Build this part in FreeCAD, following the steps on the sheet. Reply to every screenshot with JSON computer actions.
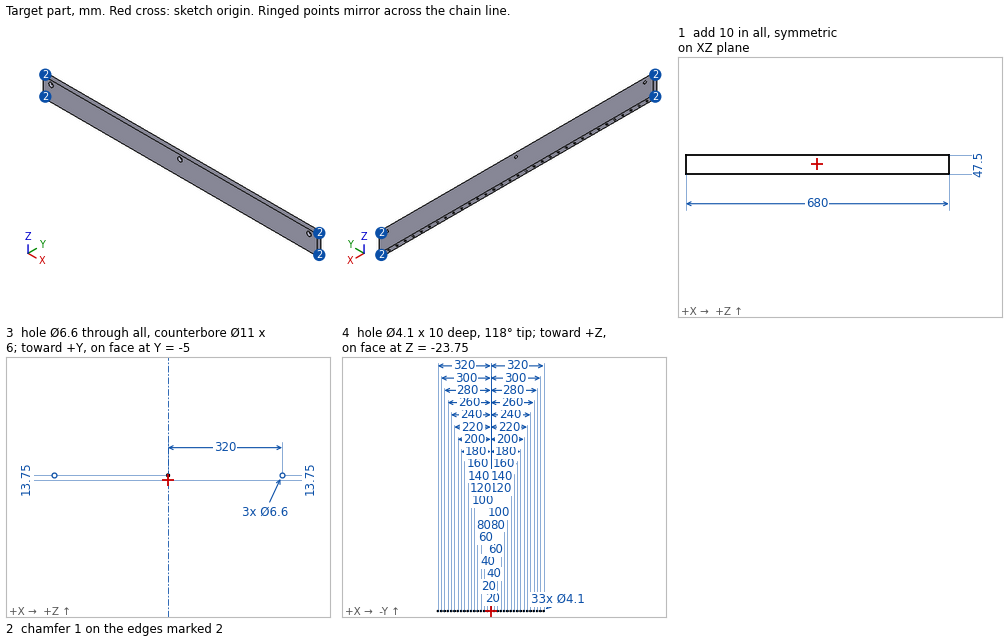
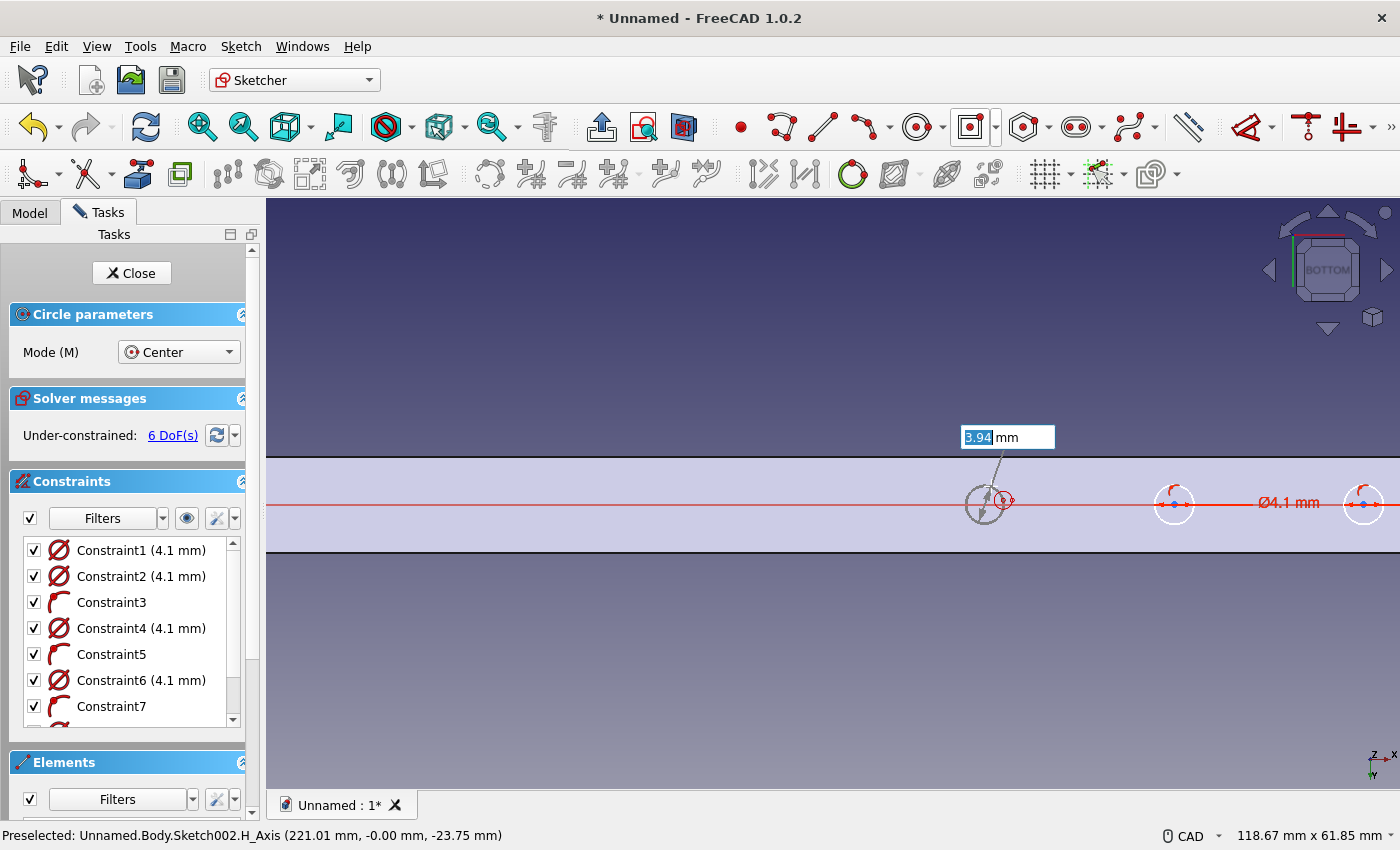
{"action": "type", "text": "4.1"}
{"action": "key", "text": "Return"}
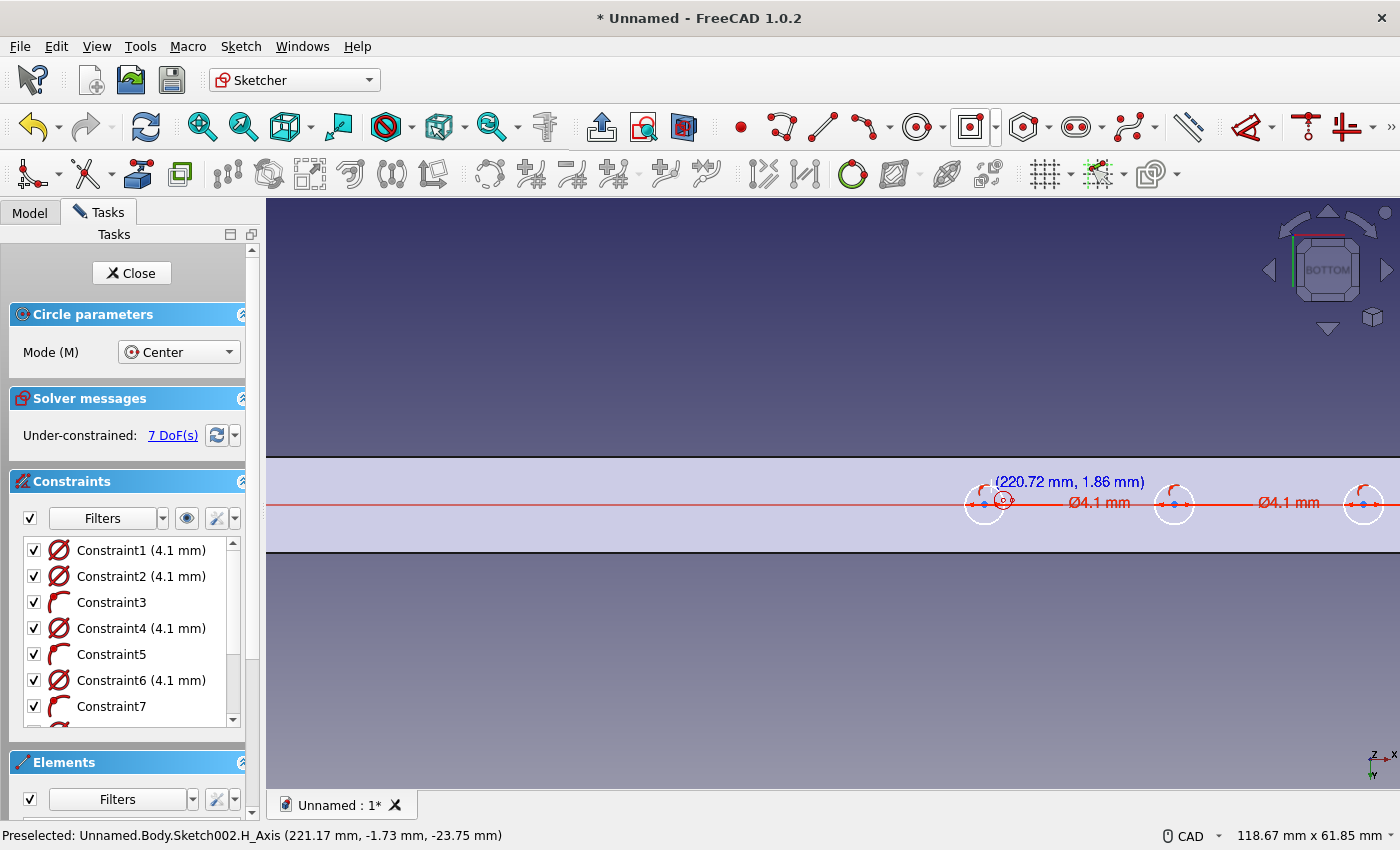
{"action": "scroll", "coordinate": [999, 492], "scroll_direction": "down", "scroll_amount": 11}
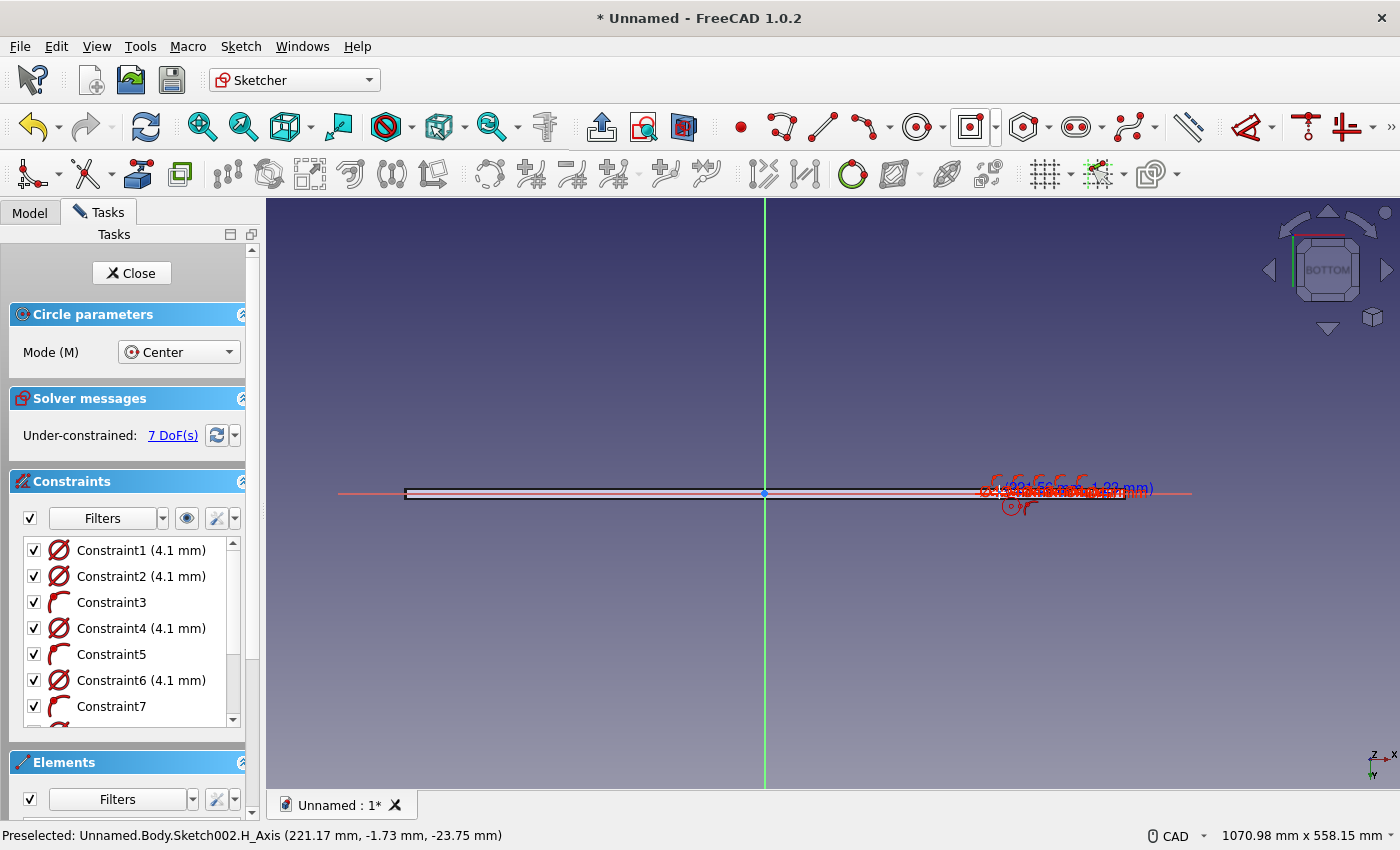
{"action": "left_click", "coordinate": [977, 494]}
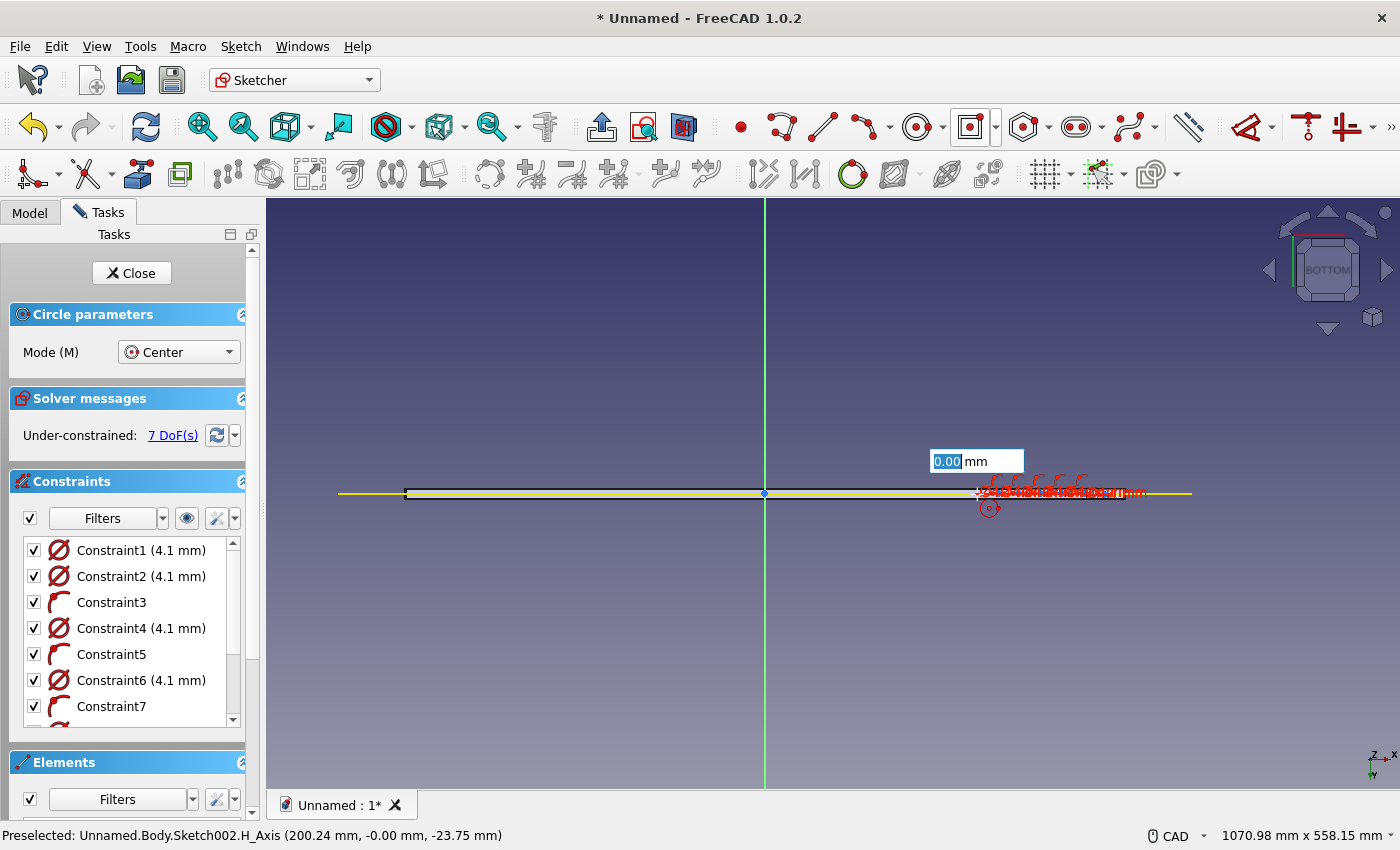
{"action": "scroll", "coordinate": [977, 492], "scroll_direction": "up", "scroll_amount": 11}
{"action": "mouse_move", "coordinate": [976, 486]}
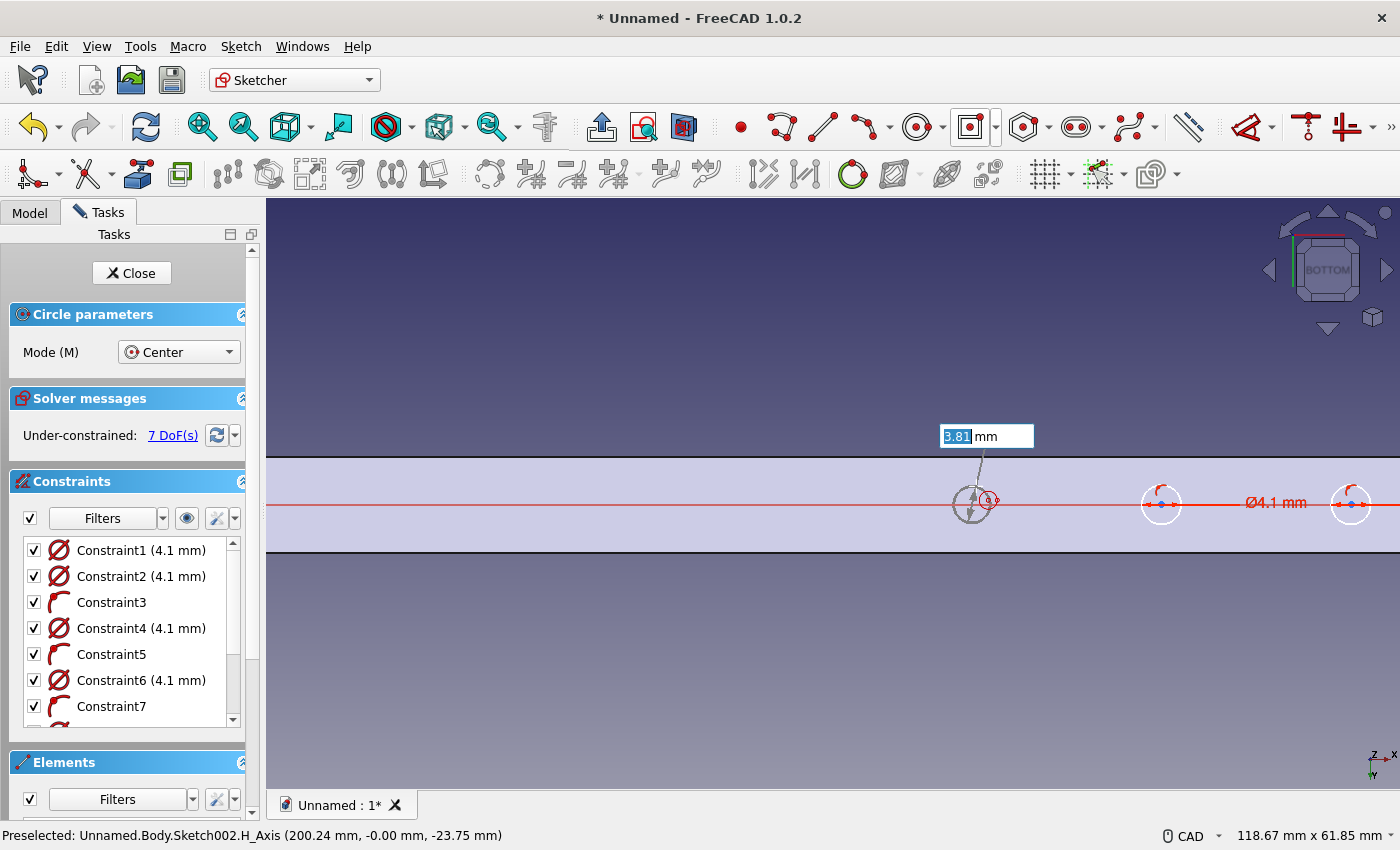
{"action": "type", "text": "4.1"}
{"action": "key", "text": "Return"}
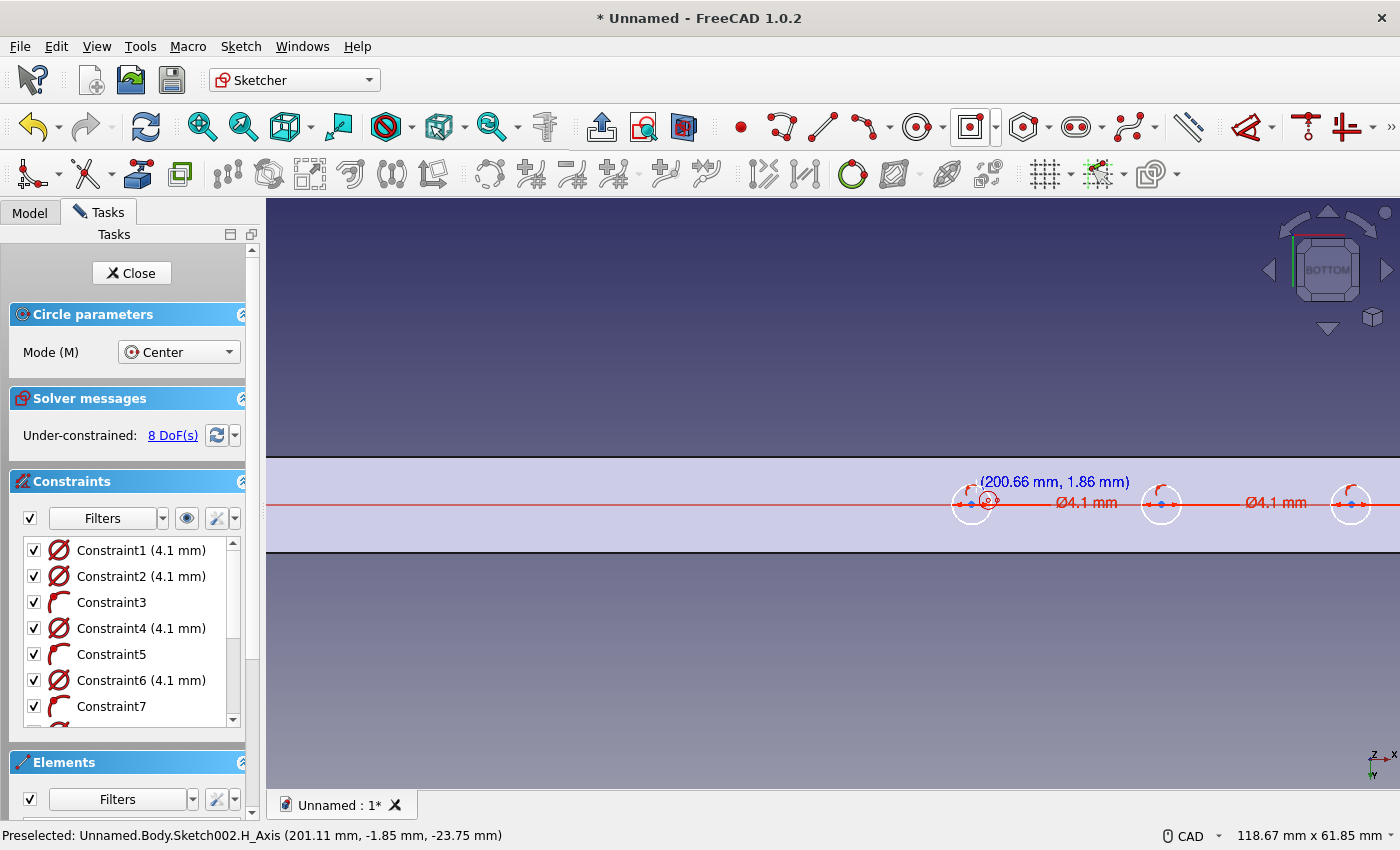
{"action": "scroll", "coordinate": [977, 492], "scroll_direction": "down", "scroll_amount": 11}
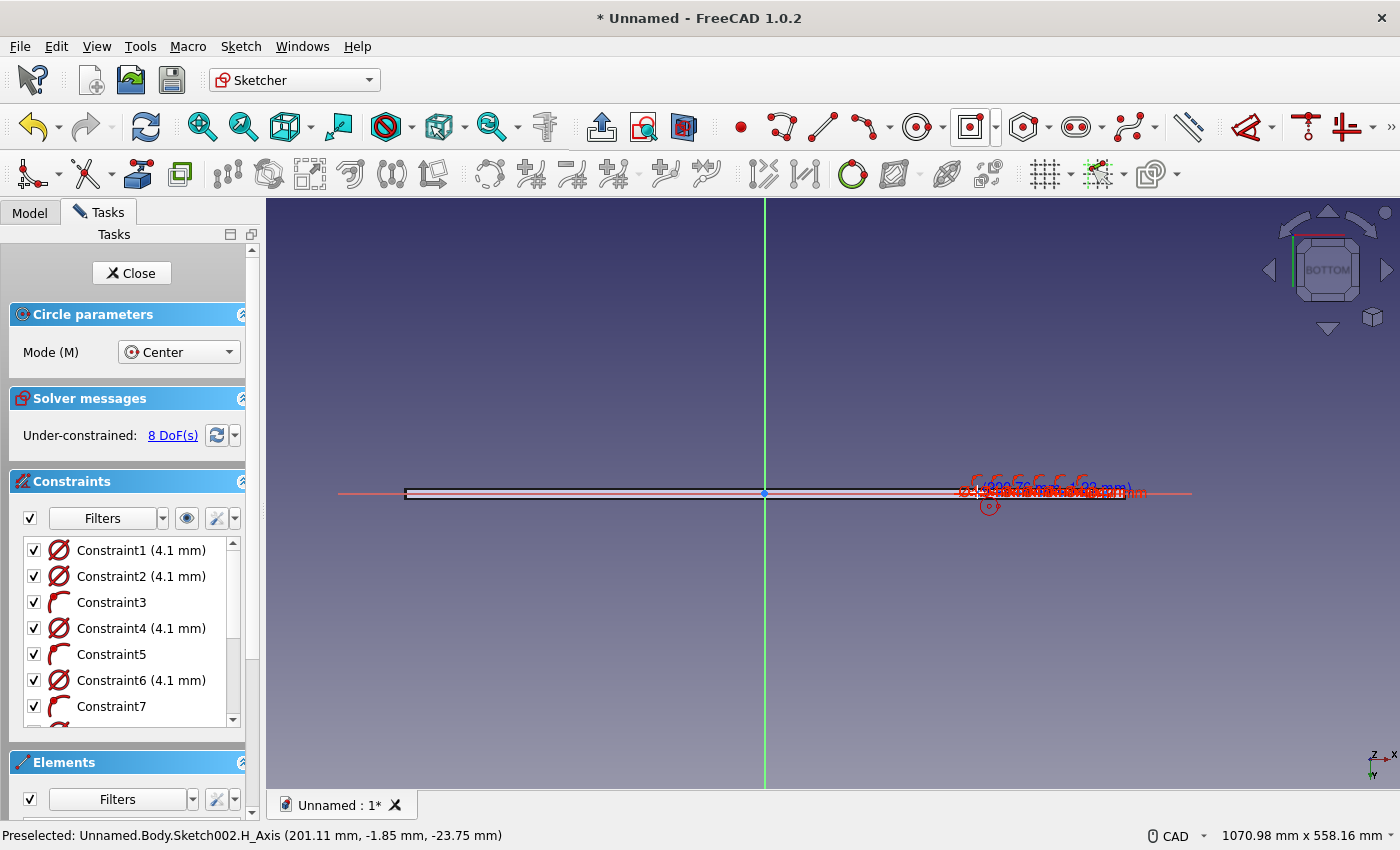
{"action": "left_click", "coordinate": [956, 494]}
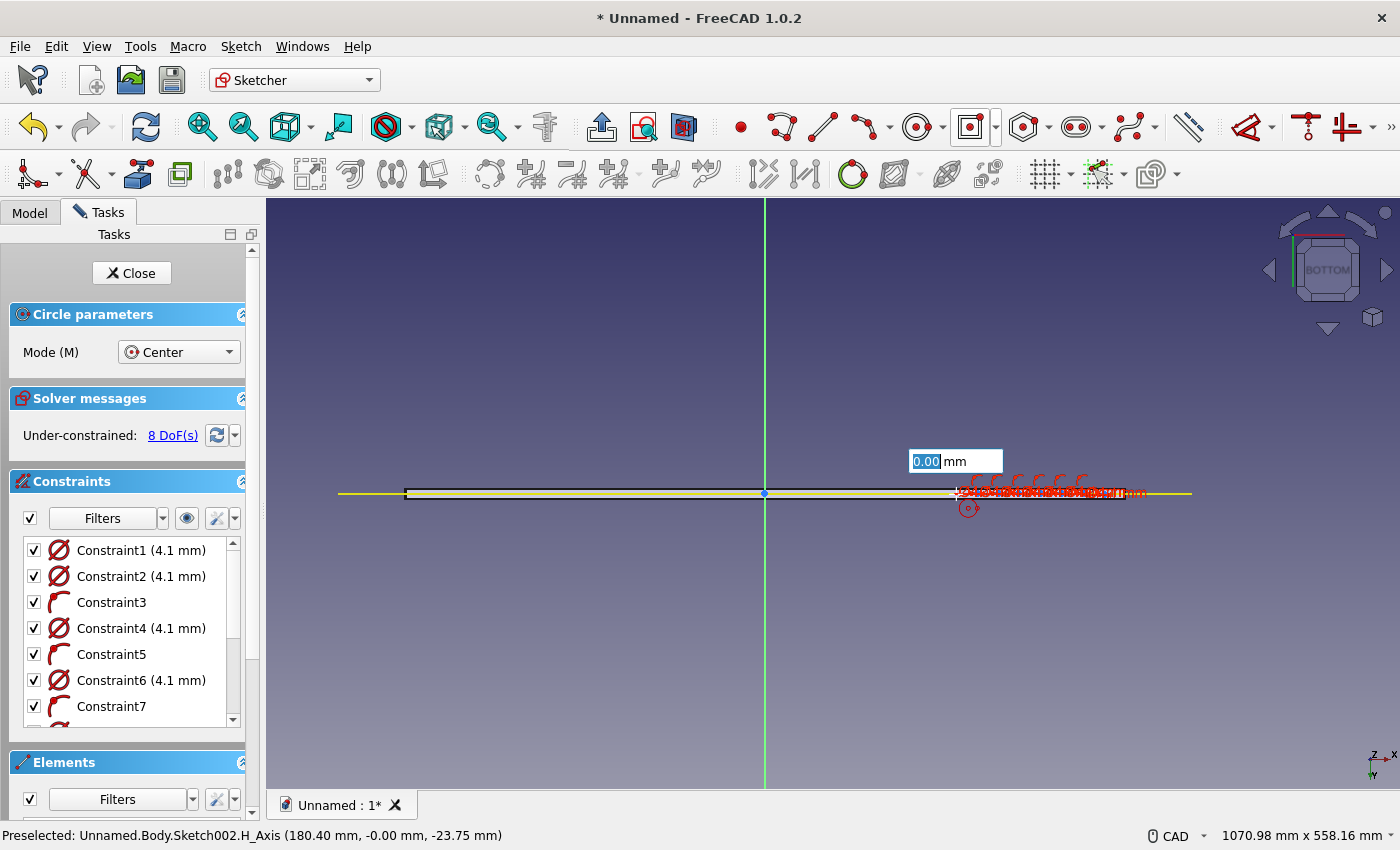
{"action": "scroll", "coordinate": [956, 492], "scroll_direction": "up", "scroll_amount": 11}
{"action": "mouse_move", "coordinate": [954, 486]}